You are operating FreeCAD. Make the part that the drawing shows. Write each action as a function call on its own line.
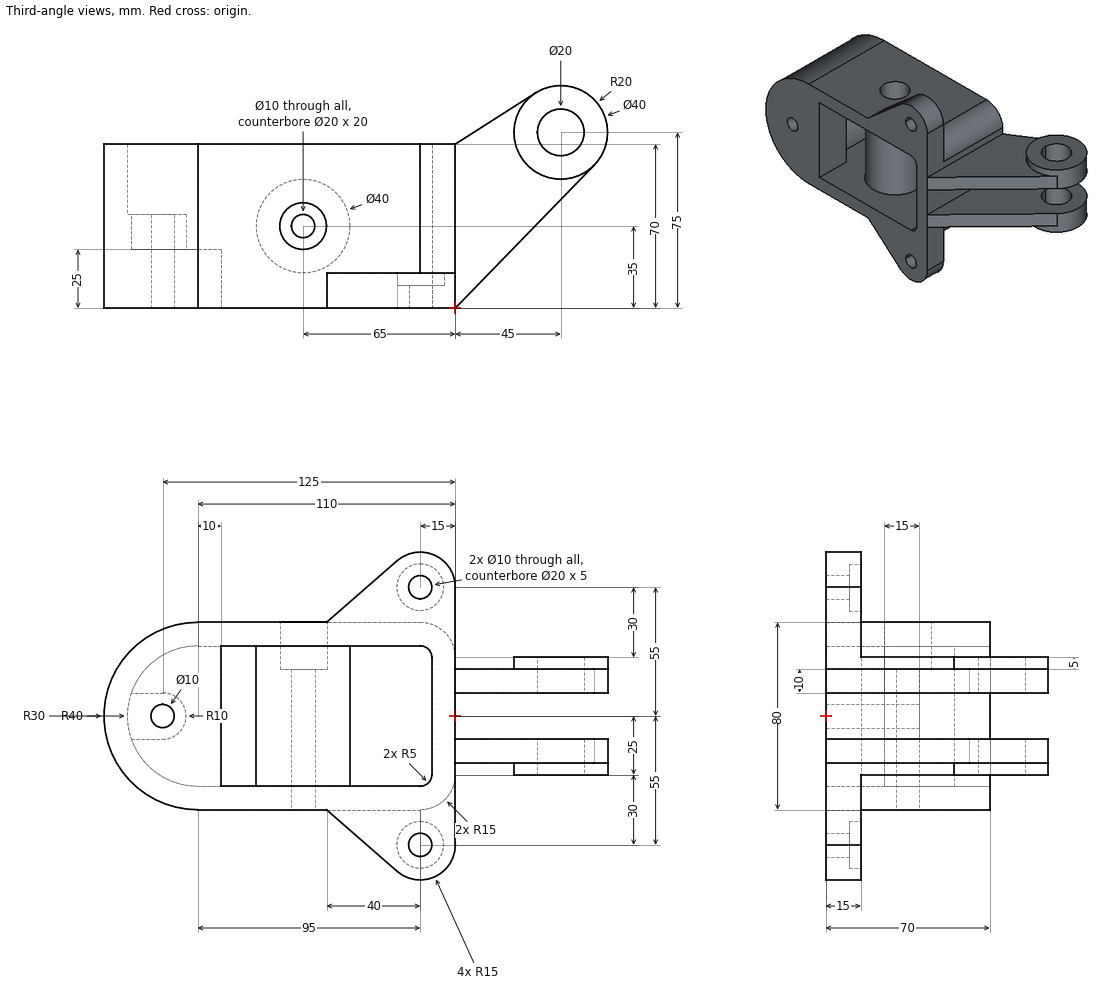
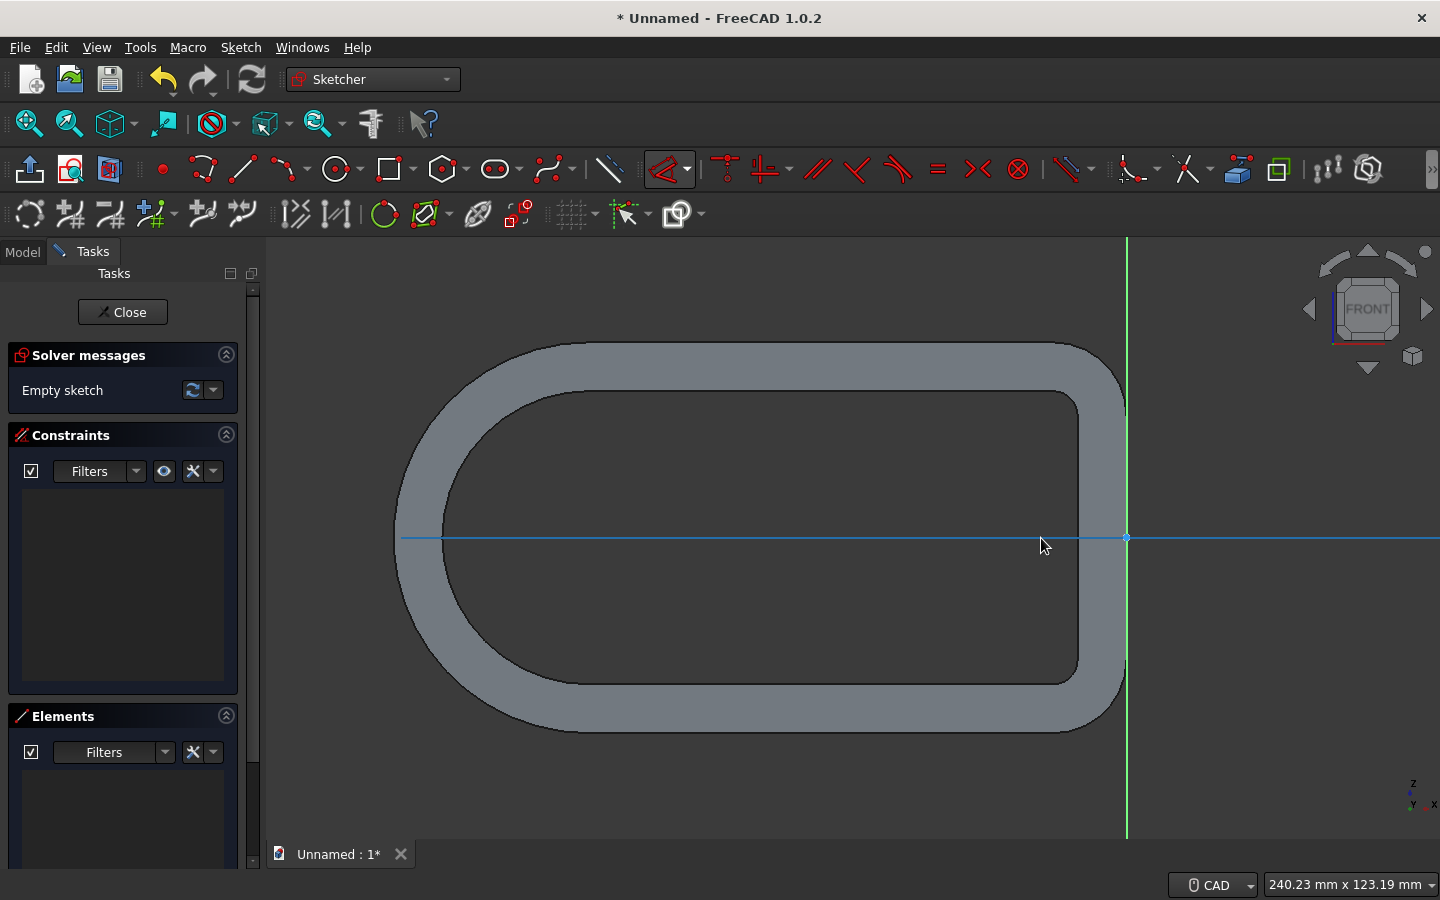
key(g)
key(m)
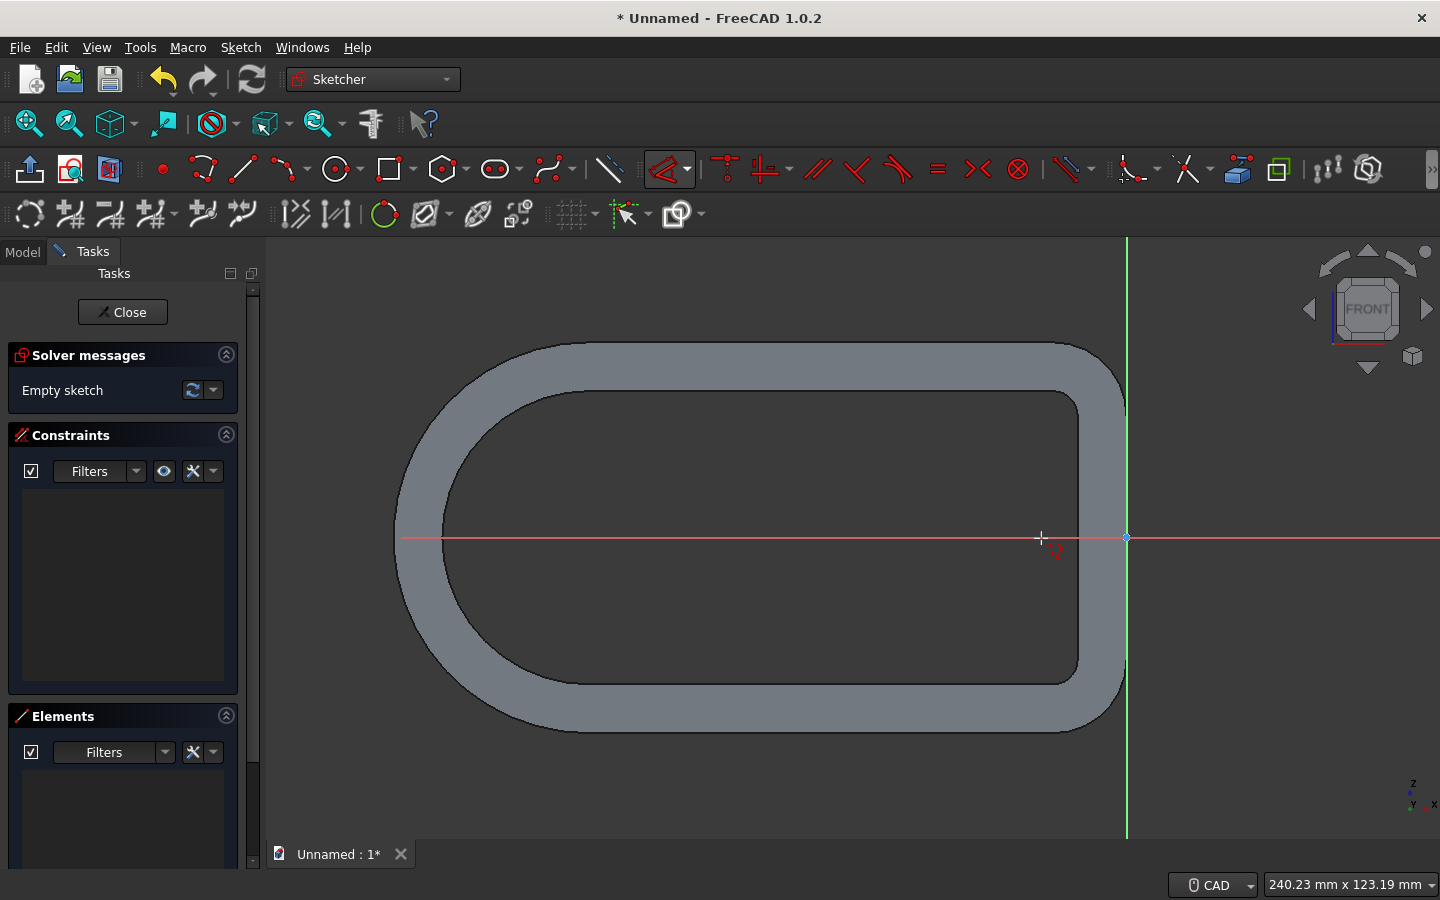
click(589, 391)
click(638, 391)
click(638, 684)
click(589, 684)
right_click(589, 684)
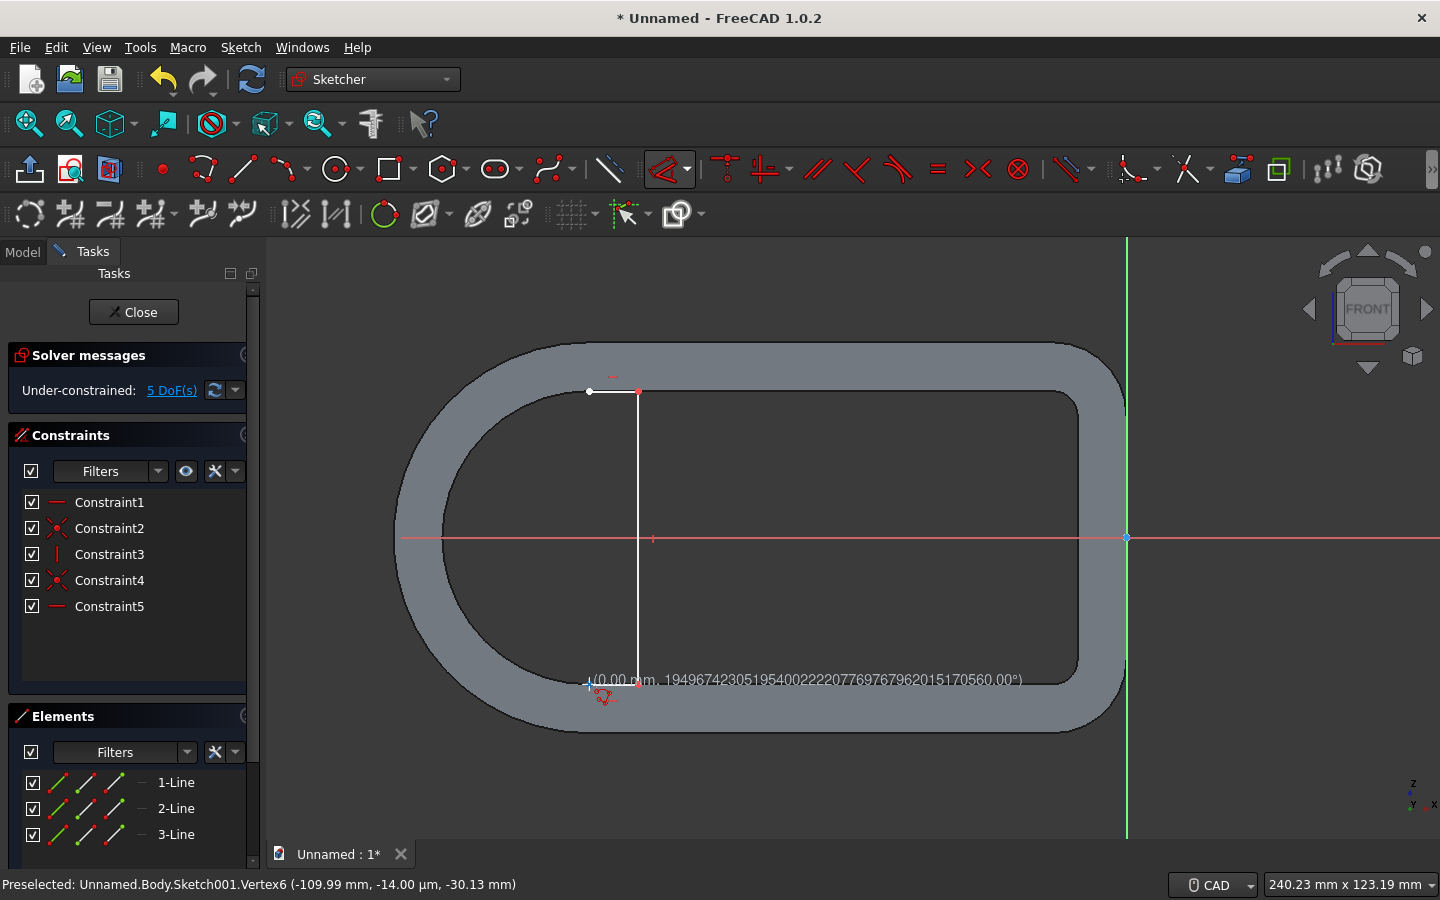
click(284, 170)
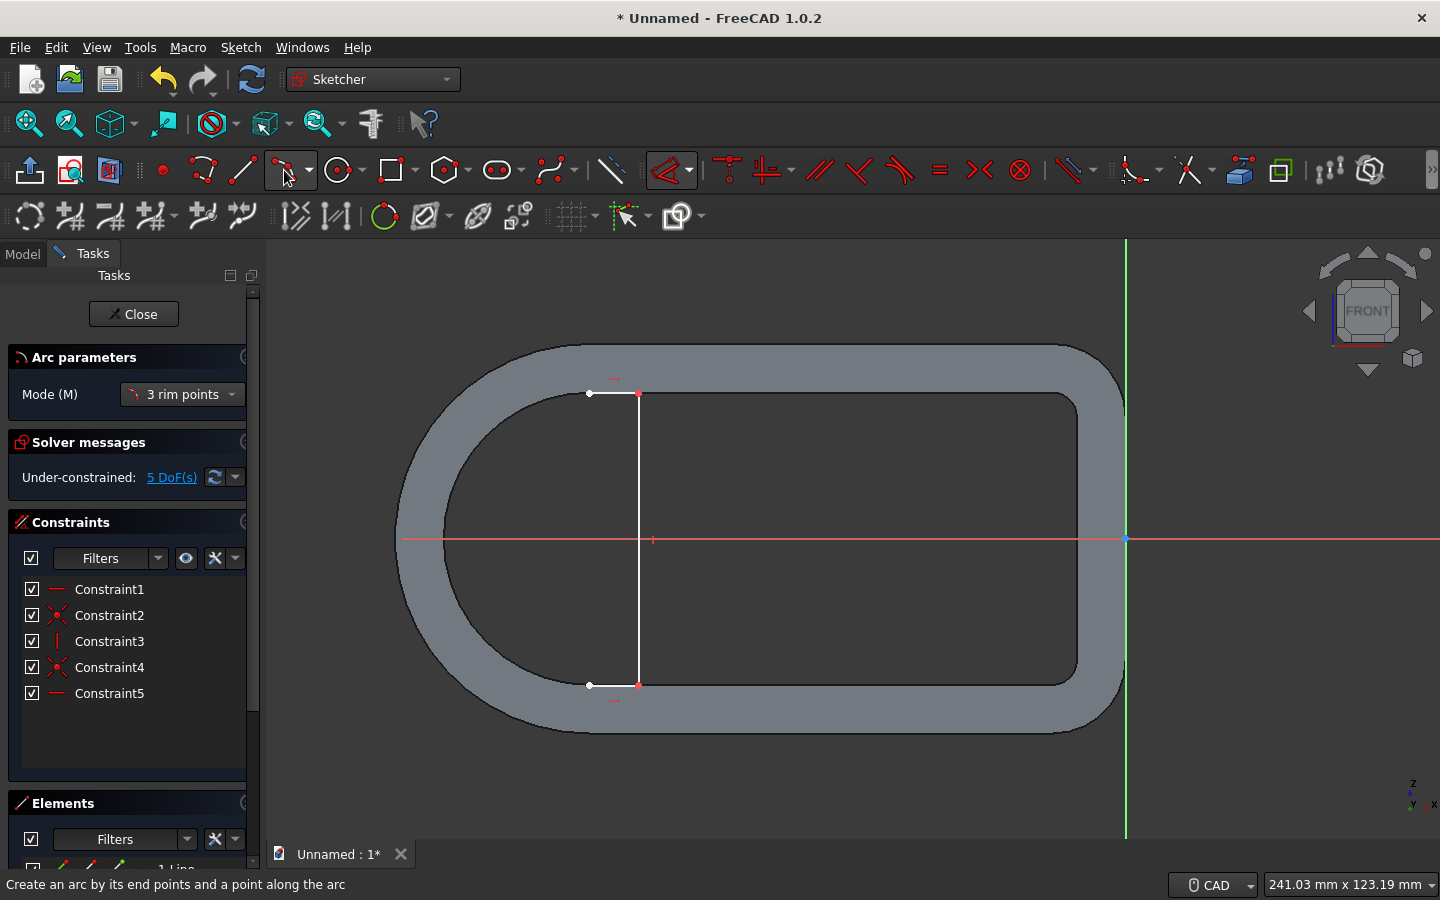
click(590, 686)
click(590, 393)
click(451, 494)
key(Escape)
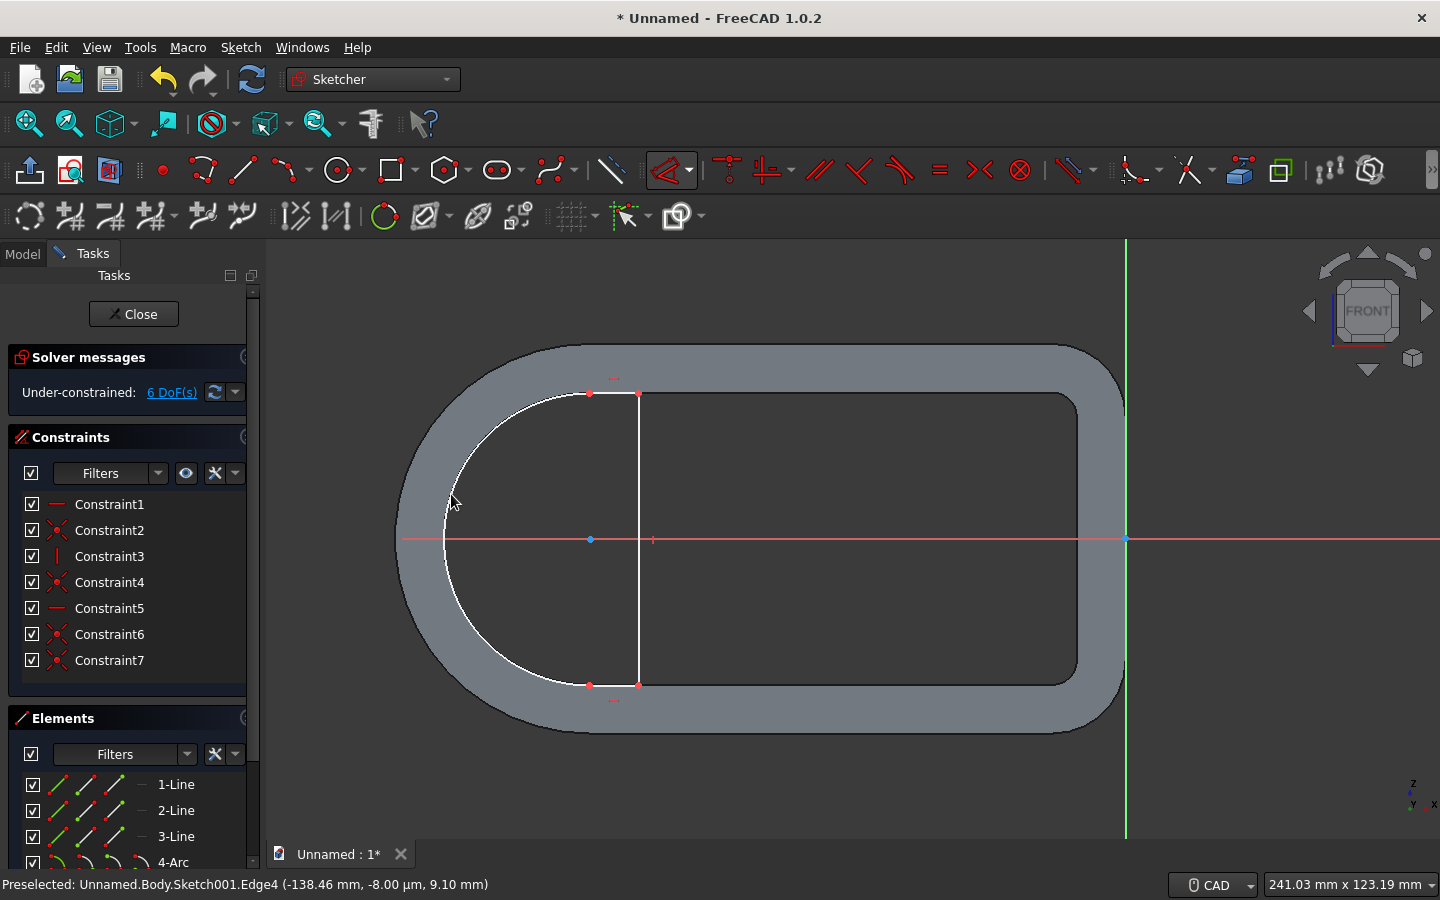
click(605, 393)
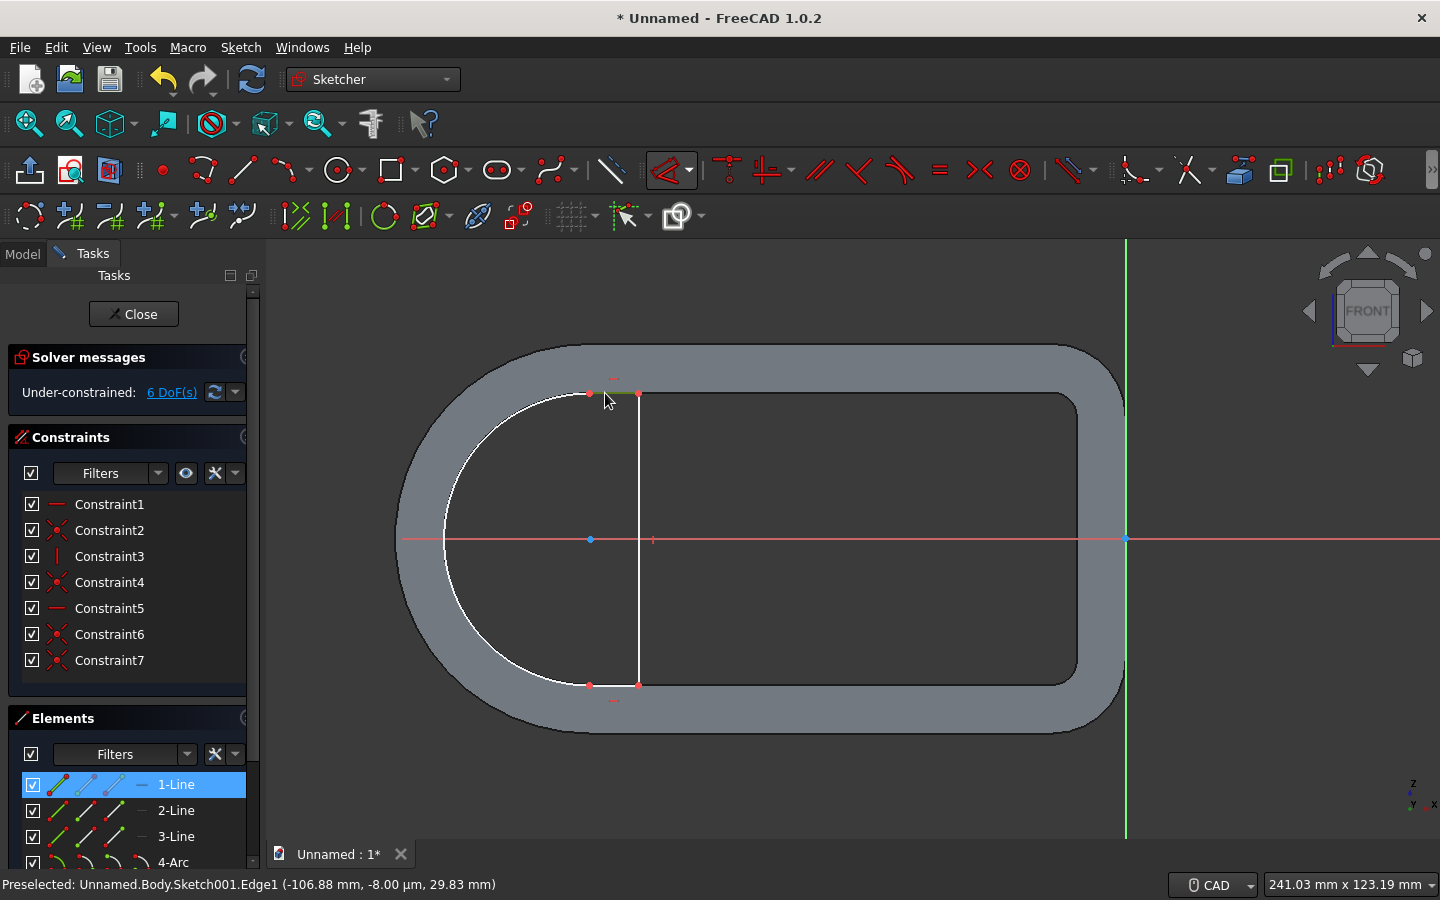
click(472, 454)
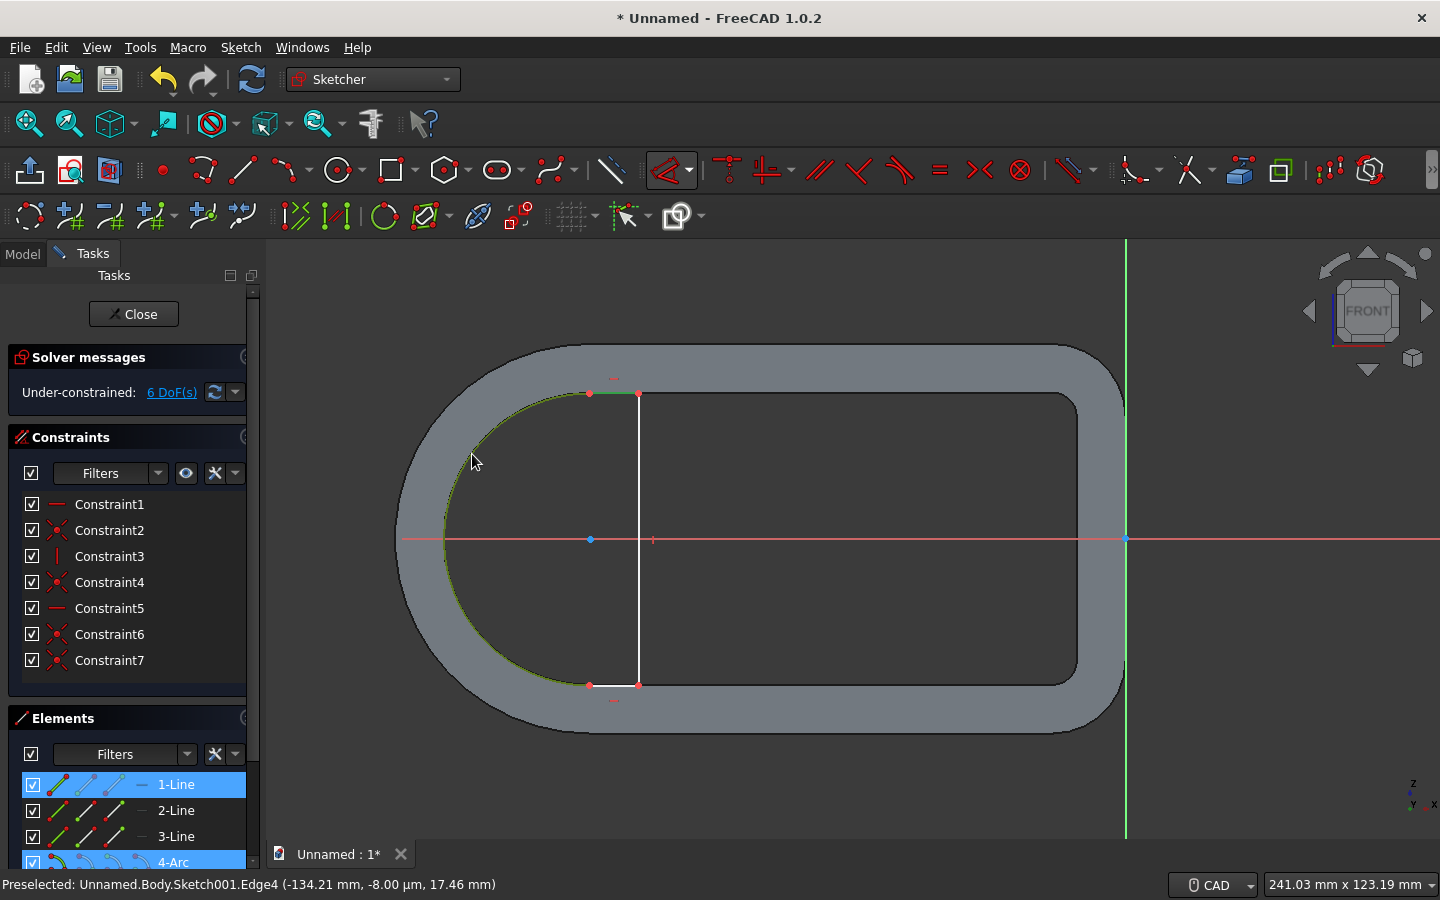
click(900, 170)